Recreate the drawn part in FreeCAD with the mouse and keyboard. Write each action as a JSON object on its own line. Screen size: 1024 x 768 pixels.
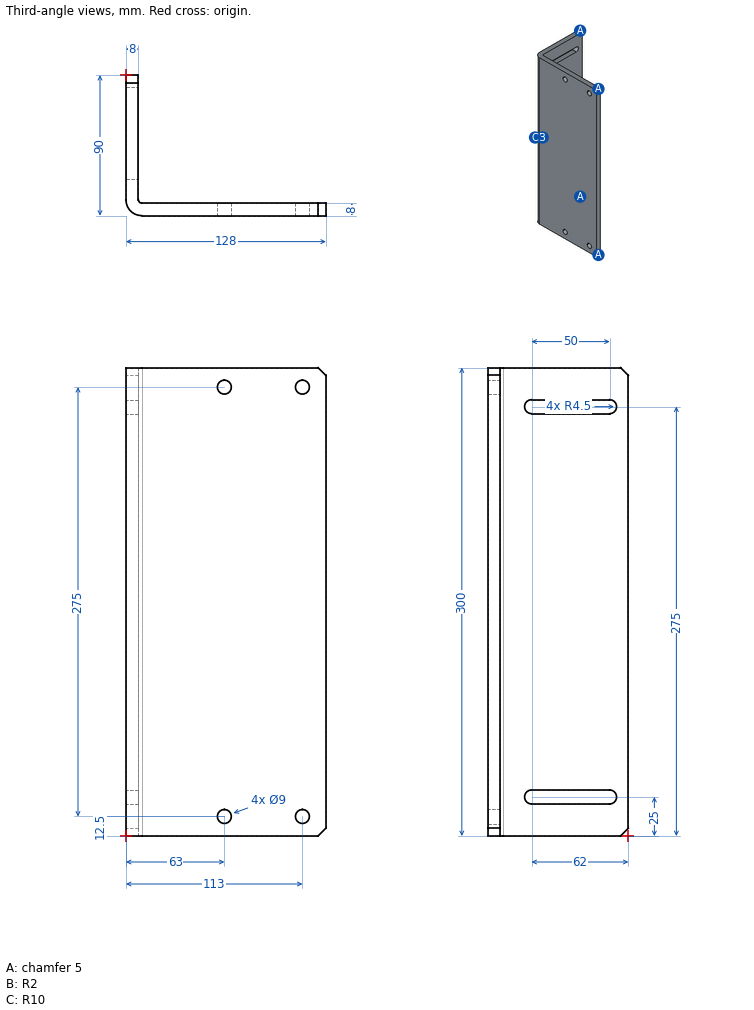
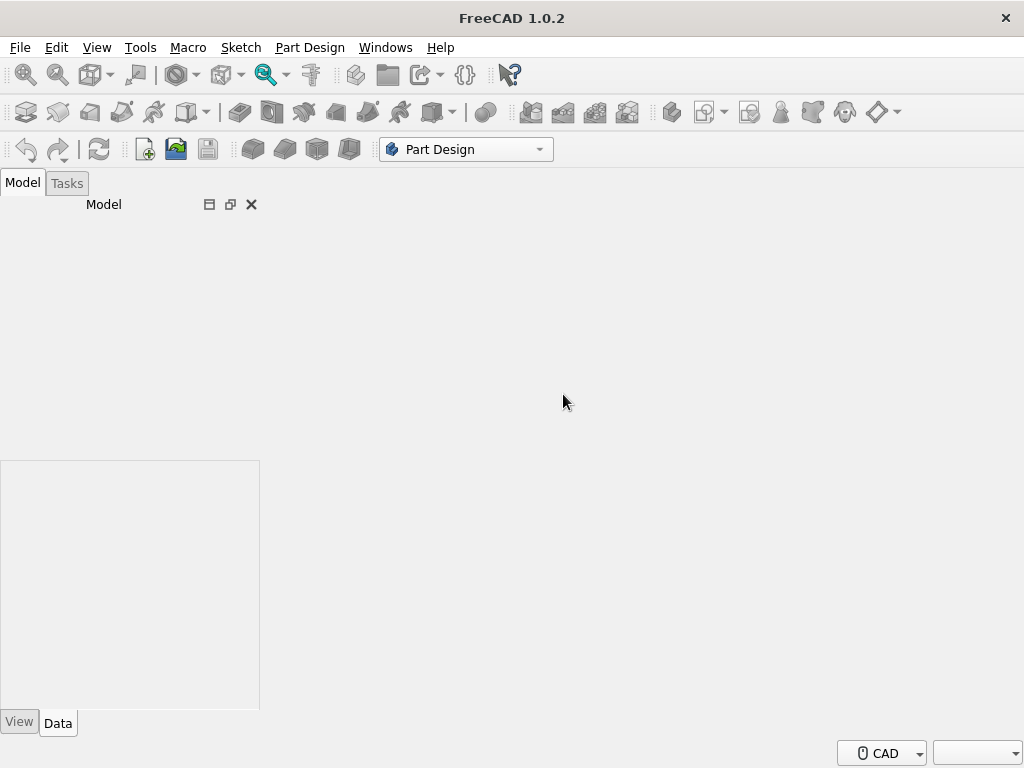
{"action": "left_click", "coordinate": [144, 150]}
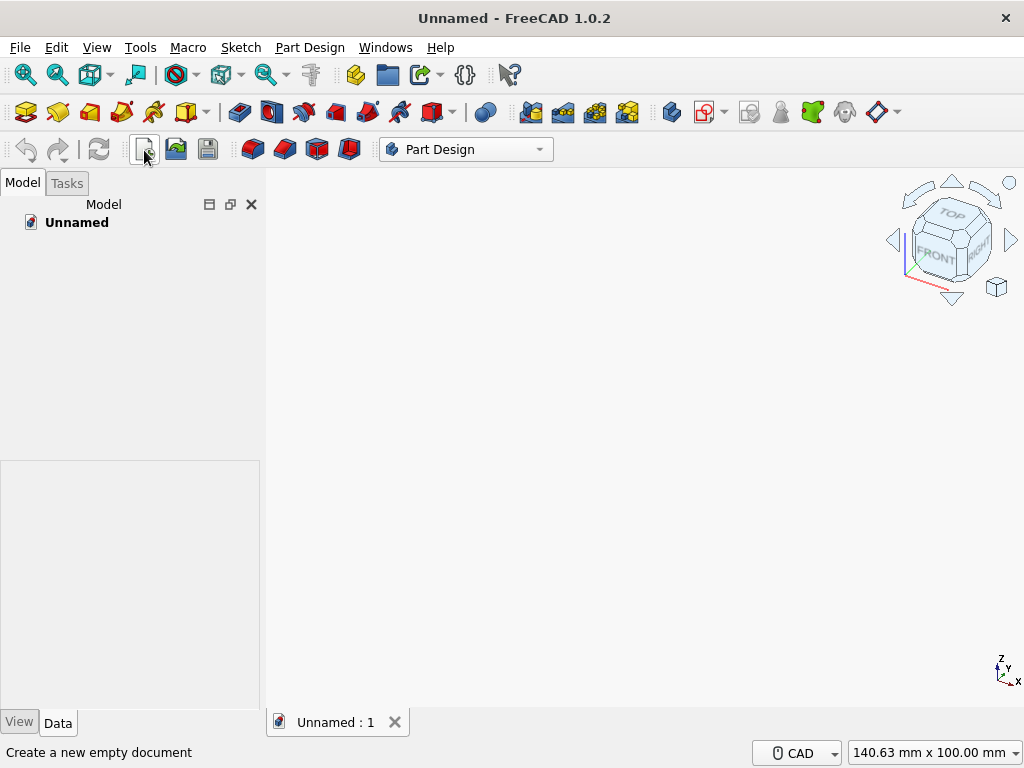
{"action": "left_click", "coordinate": [704, 112]}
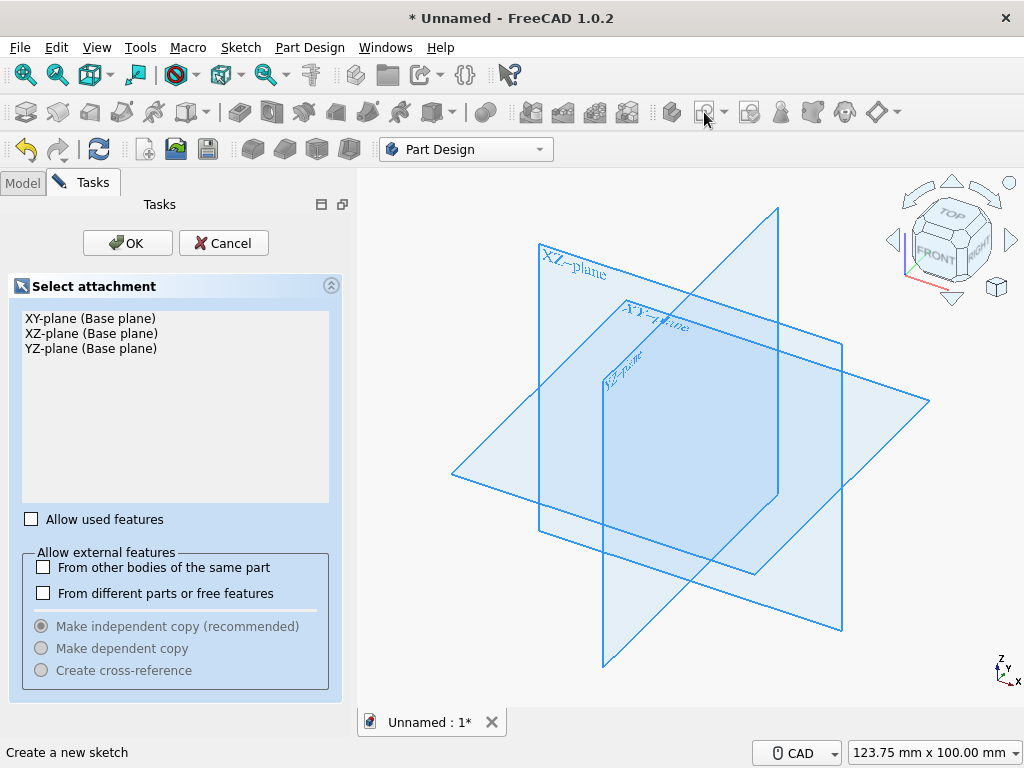
{"action": "left_click", "coordinate": [82, 318]}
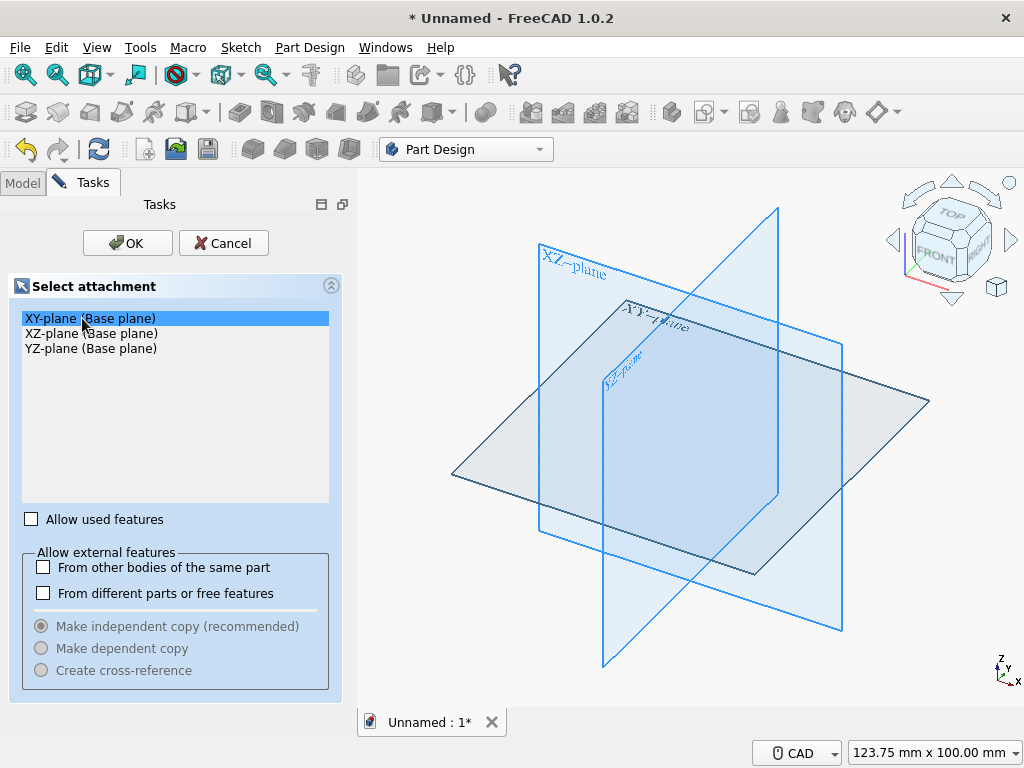
{"action": "left_click", "coordinate": [128, 243]}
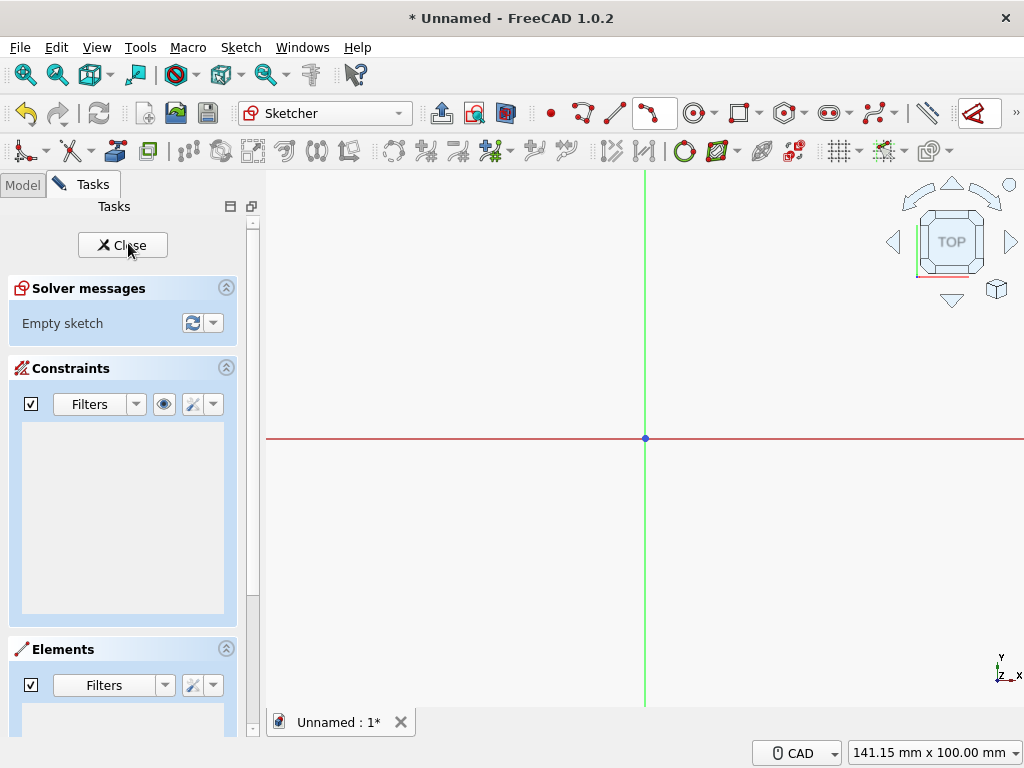
{"action": "scroll", "coordinate": [294, 241], "scroll_direction": "down", "scroll_amount": 4}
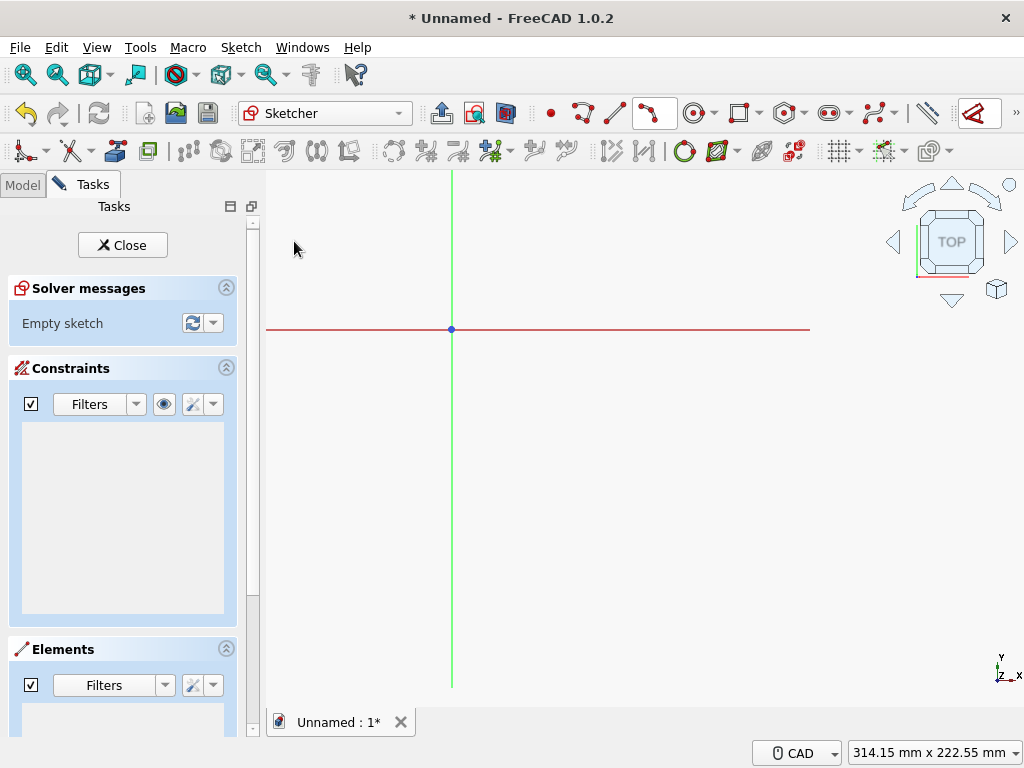
{"action": "left_click", "coordinate": [584, 114]}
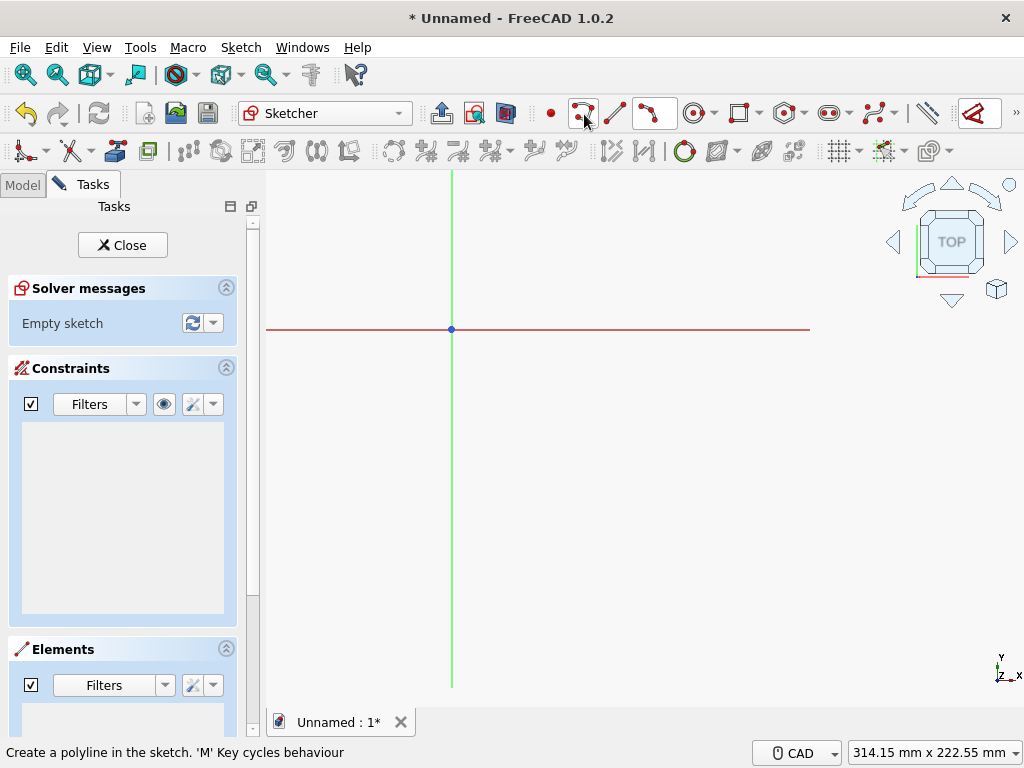
{"action": "left_click", "coordinate": [452, 330]}
{"action": "left_click", "coordinate": [461, 547]}
{"action": "left_click", "coordinate": [761, 547]}
{"action": "left_click", "coordinate": [761, 528]}
{"action": "left_click", "coordinate": [471, 528]}
{"action": "left_click", "coordinate": [471, 339]}
{"action": "left_click", "coordinate": [452, 330]}
{"action": "key", "text": "Escape"}
{"action": "key", "text": "Escape"}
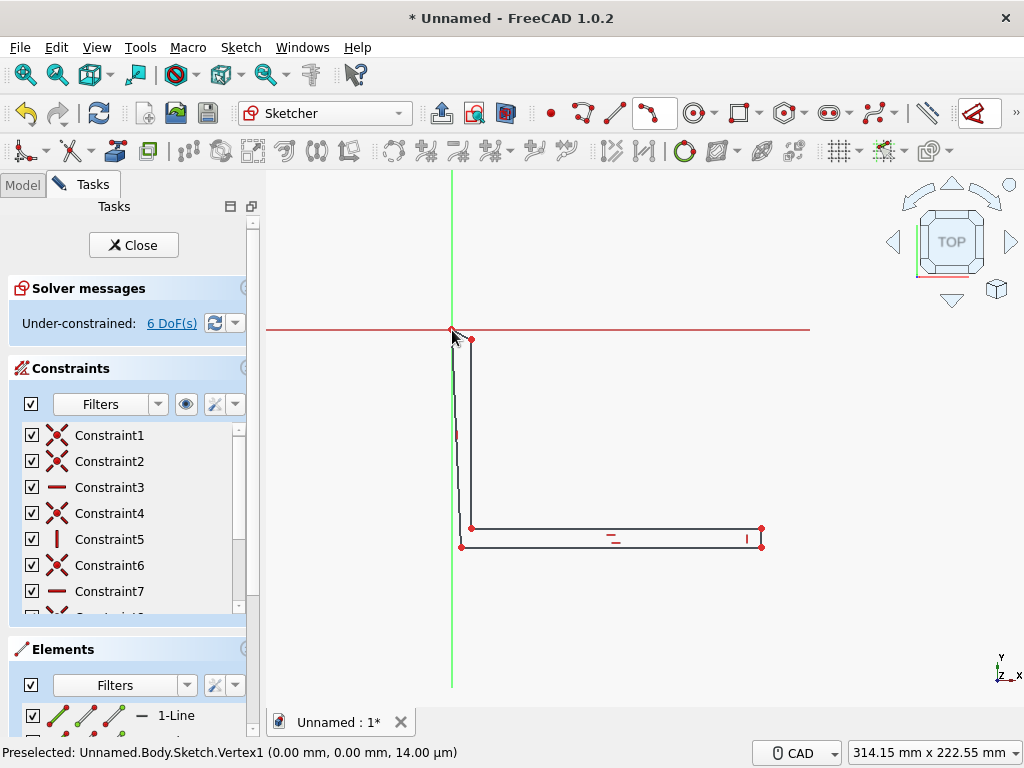
{"action": "left_click", "coordinate": [455, 395]}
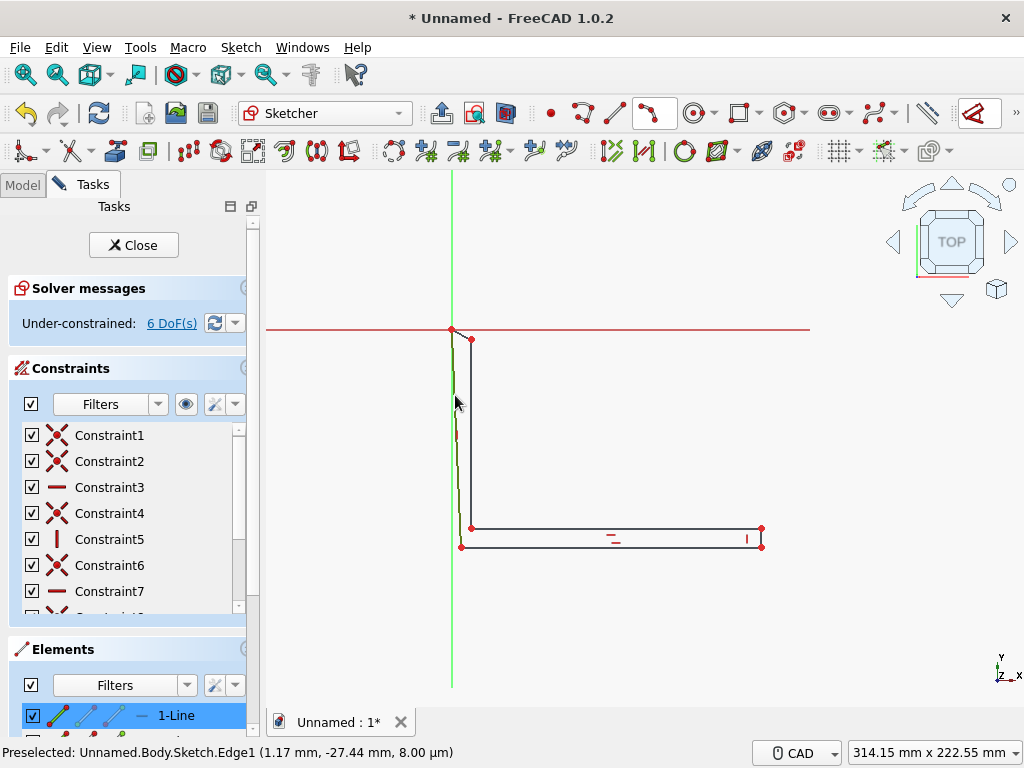
{"action": "key", "text": "v"}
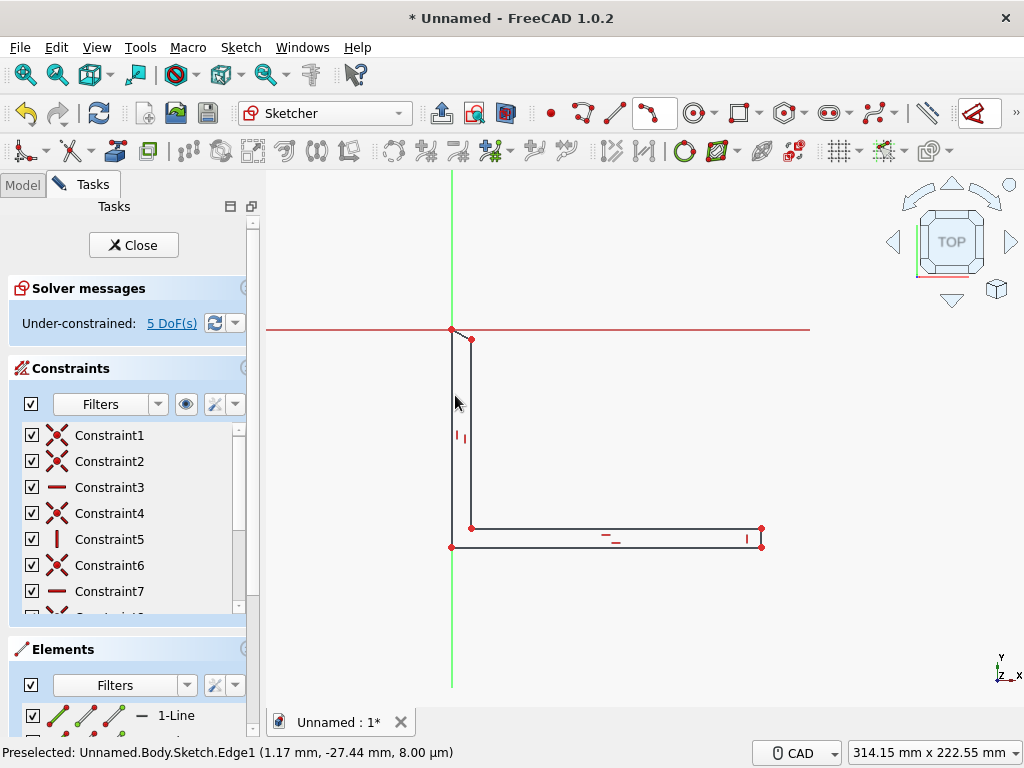
{"action": "scroll", "coordinate": [465, 337], "scroll_direction": "up", "scroll_amount": 4}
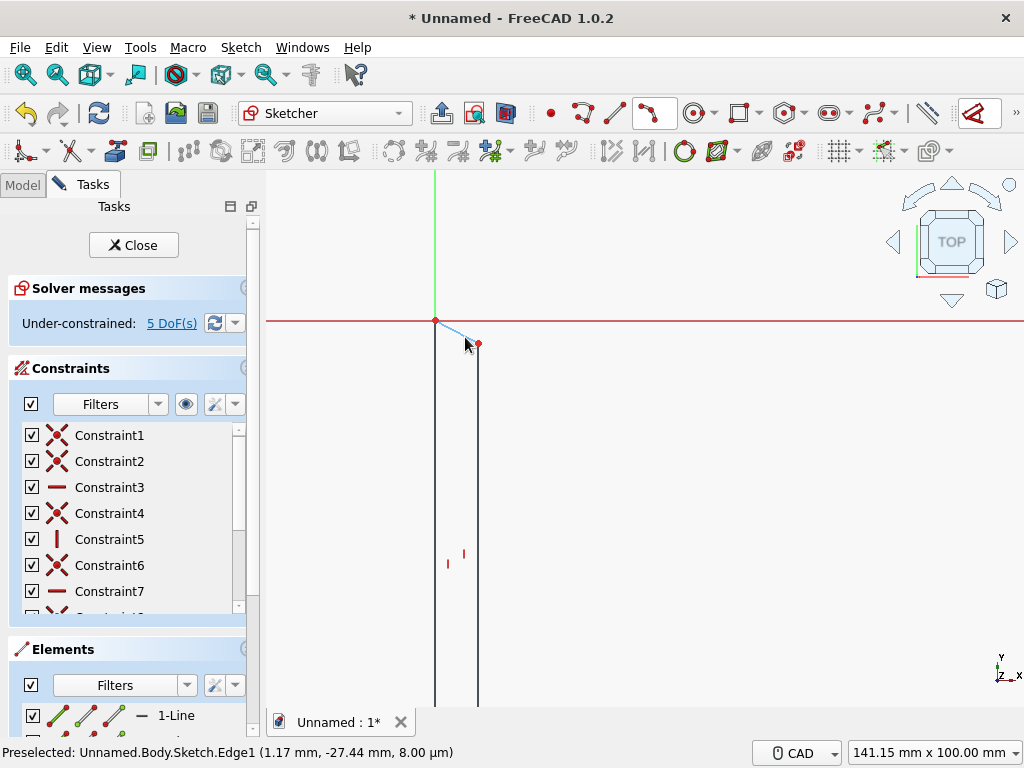
{"action": "left_click", "coordinate": [465, 336]}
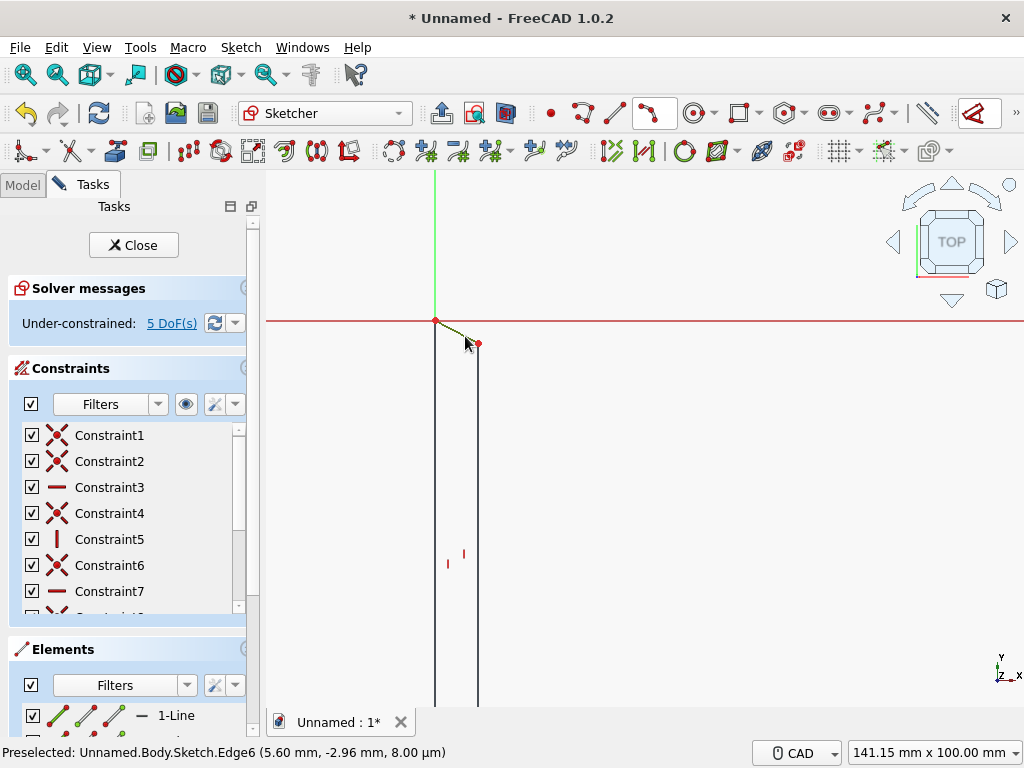
{"action": "key", "text": "h"}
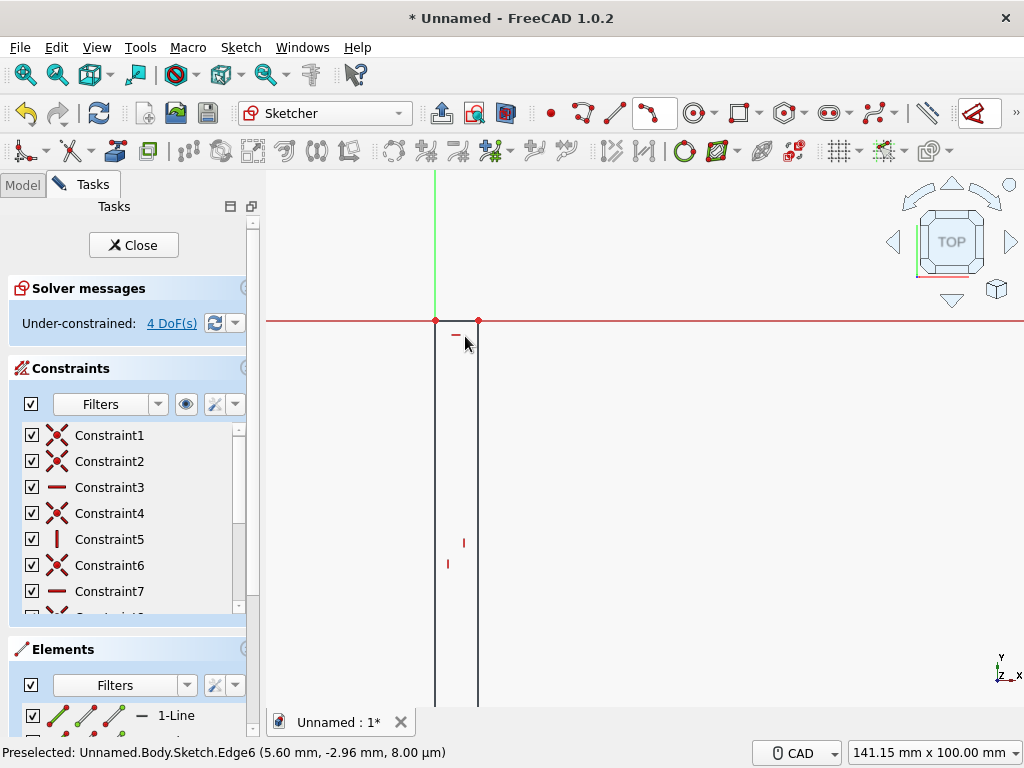
{"action": "key", "text": "d"}